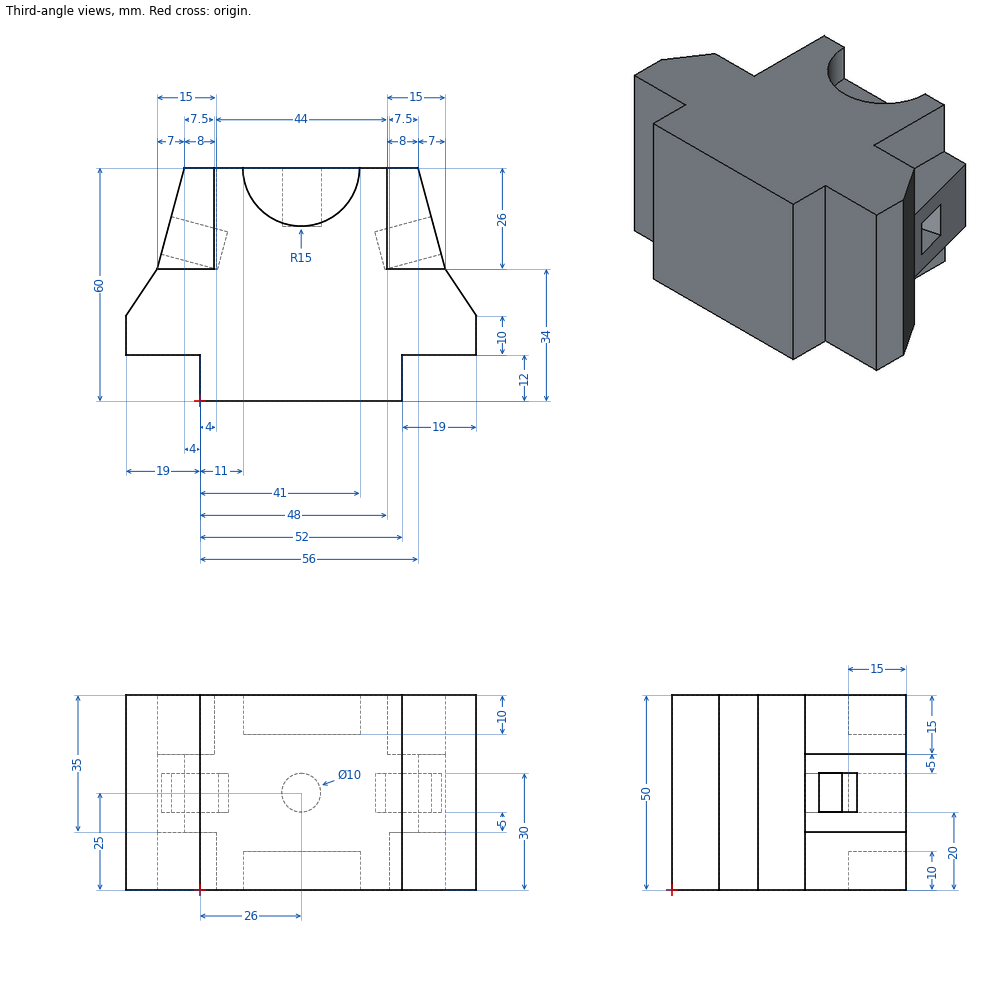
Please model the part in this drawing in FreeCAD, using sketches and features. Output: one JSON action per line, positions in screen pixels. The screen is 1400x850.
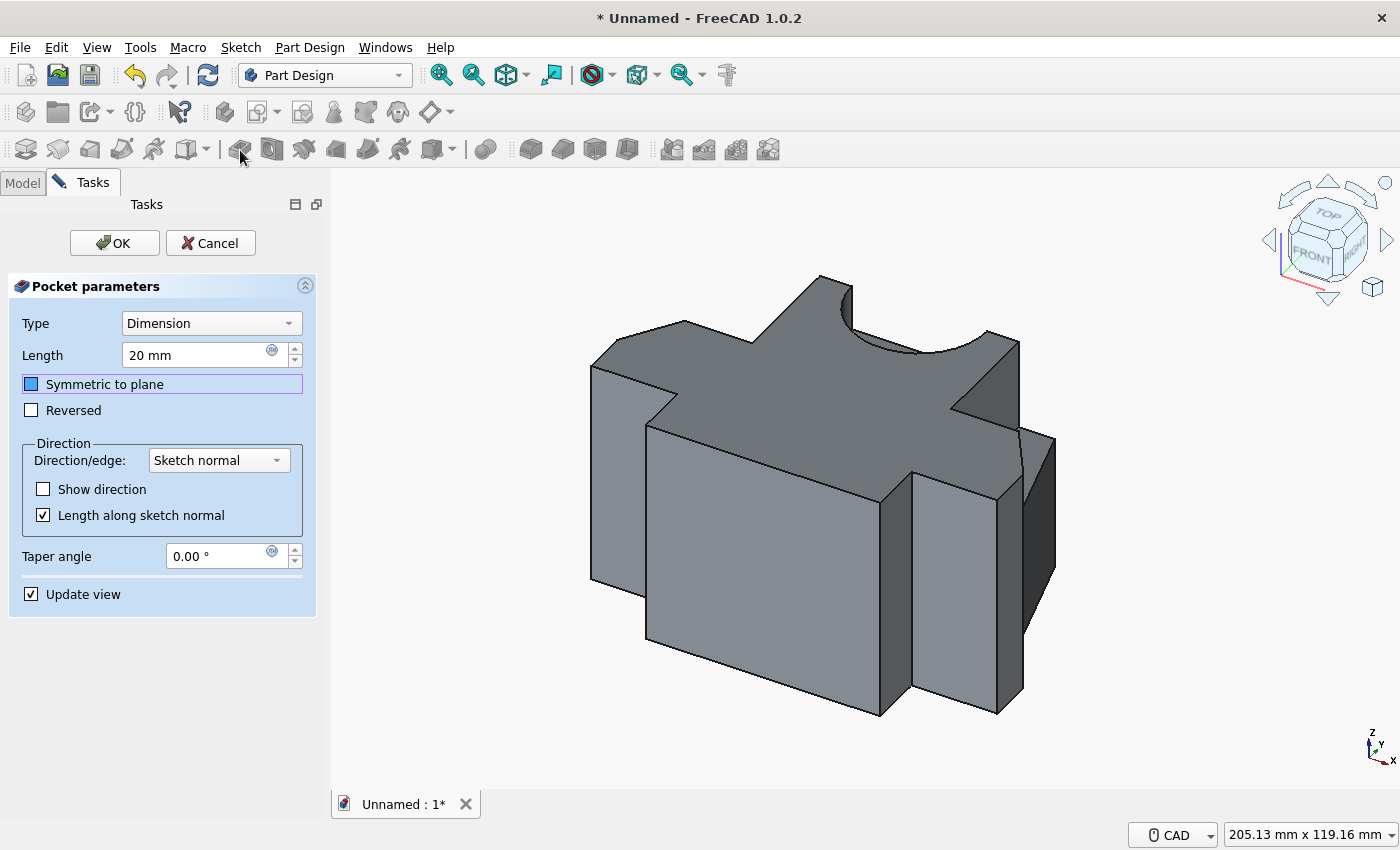
{"action": "left_click", "coordinate": [30, 410]}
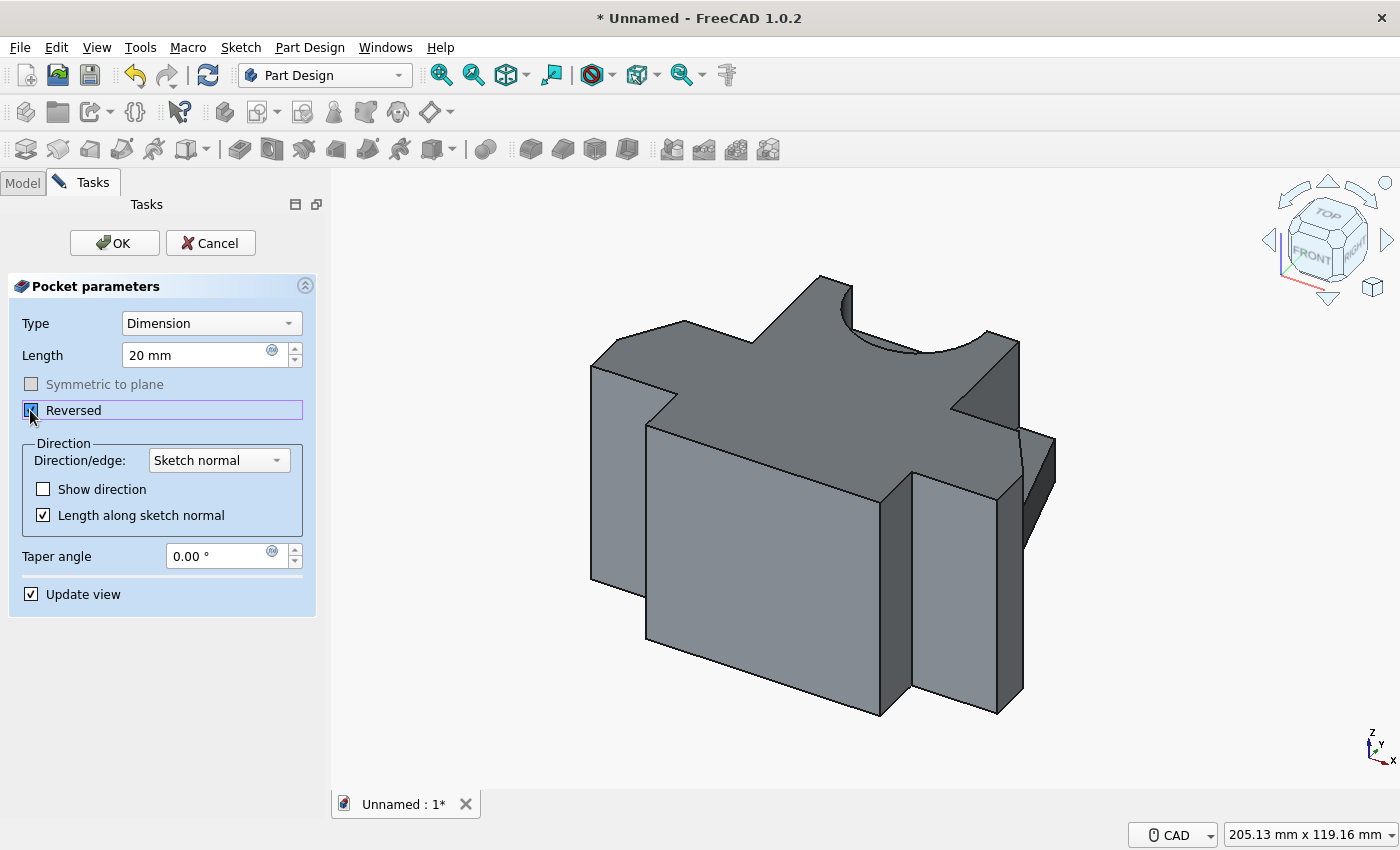
{"action": "left_click", "coordinate": [115, 243]}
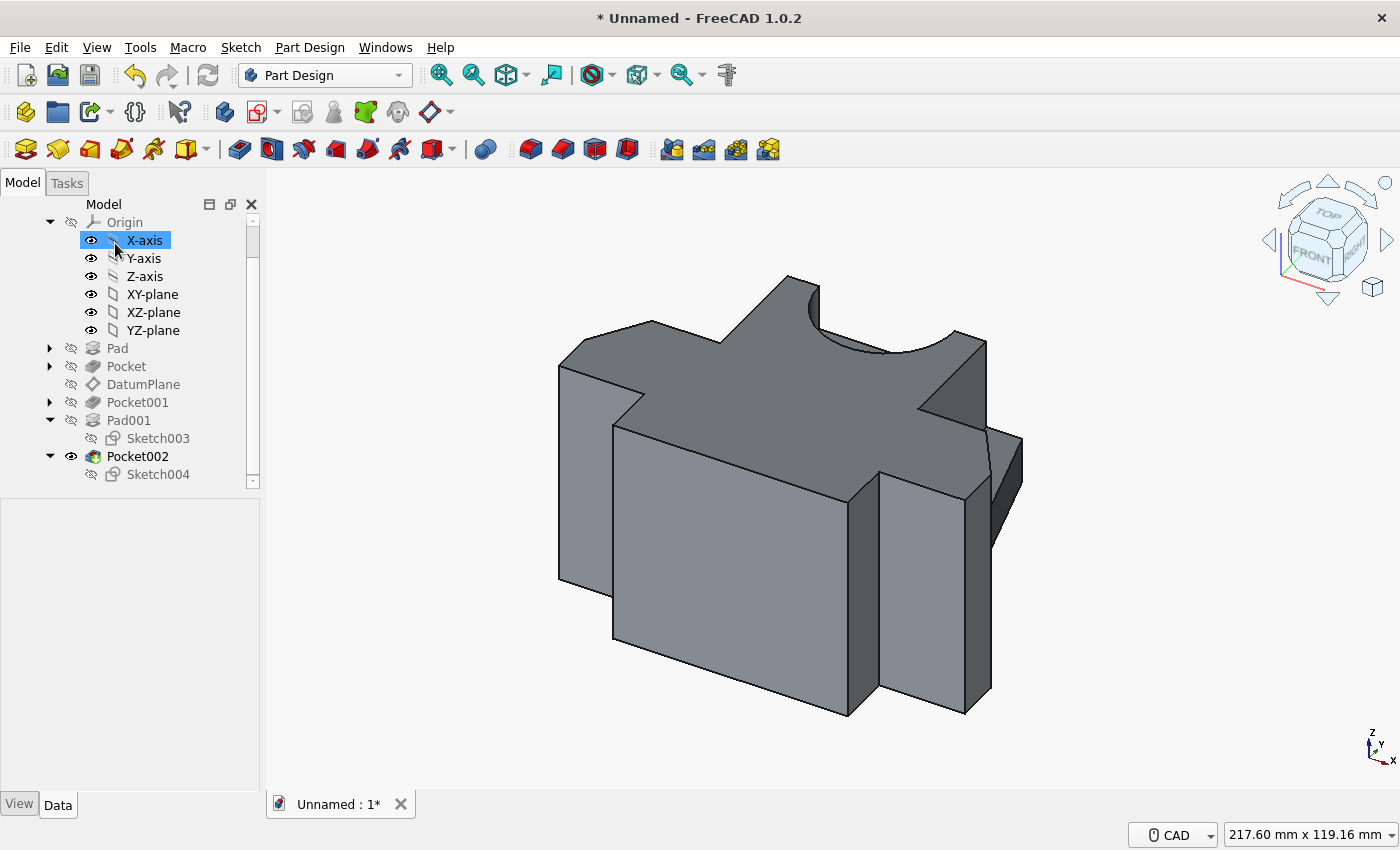
{"action": "key", "text": "5"}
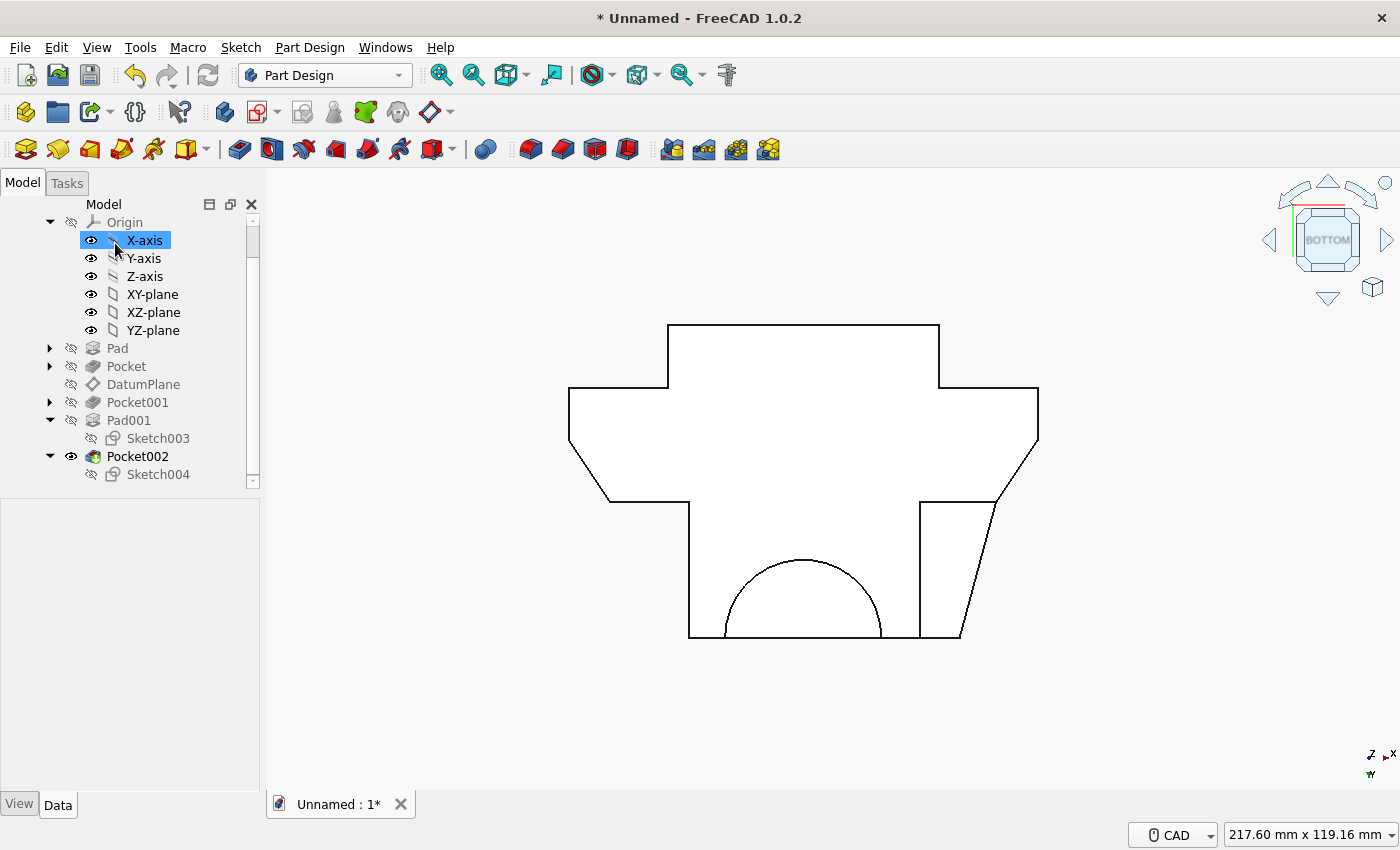
{"action": "left_click", "coordinate": [958, 530]}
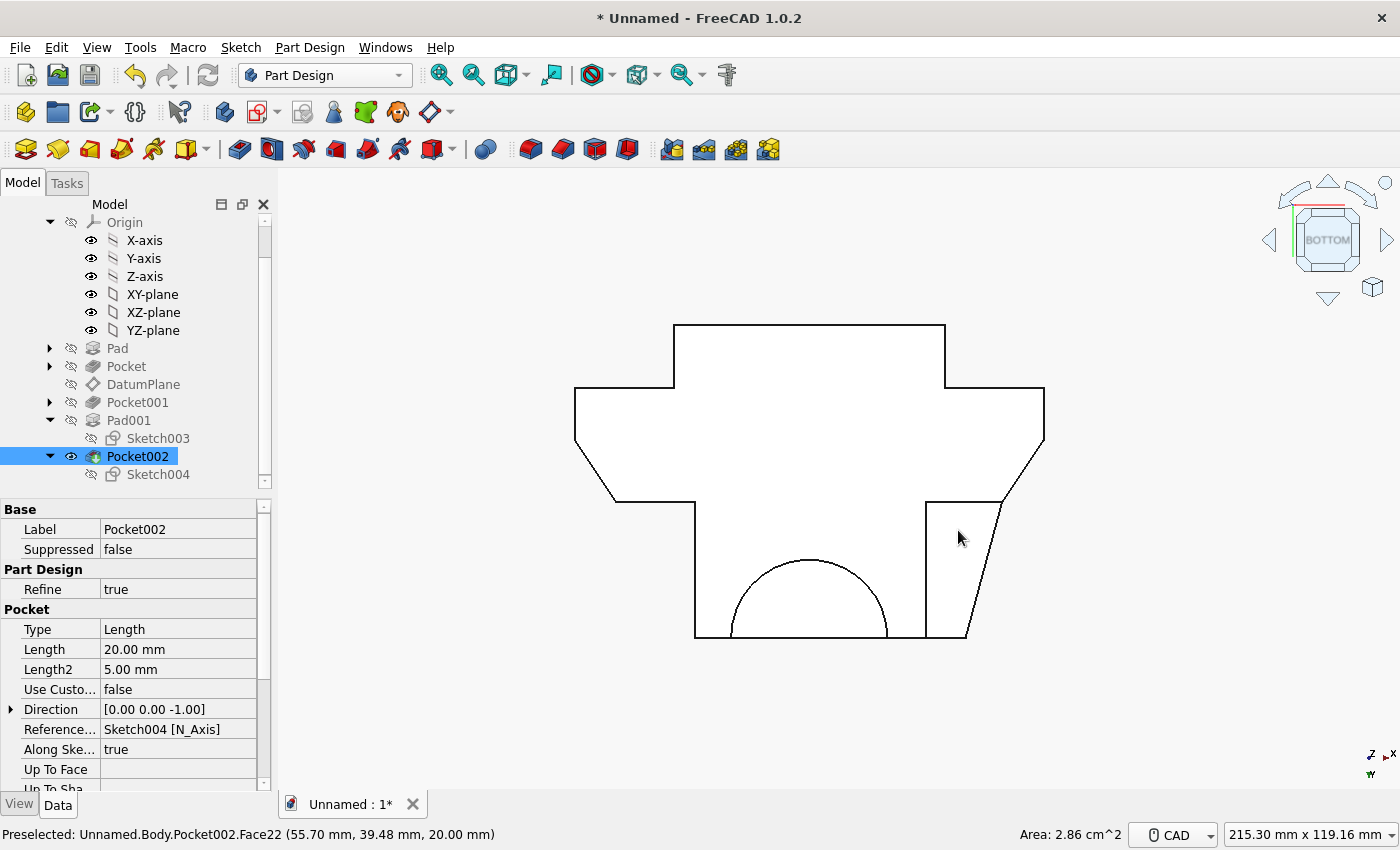
{"action": "left_click", "coordinate": [258, 112]}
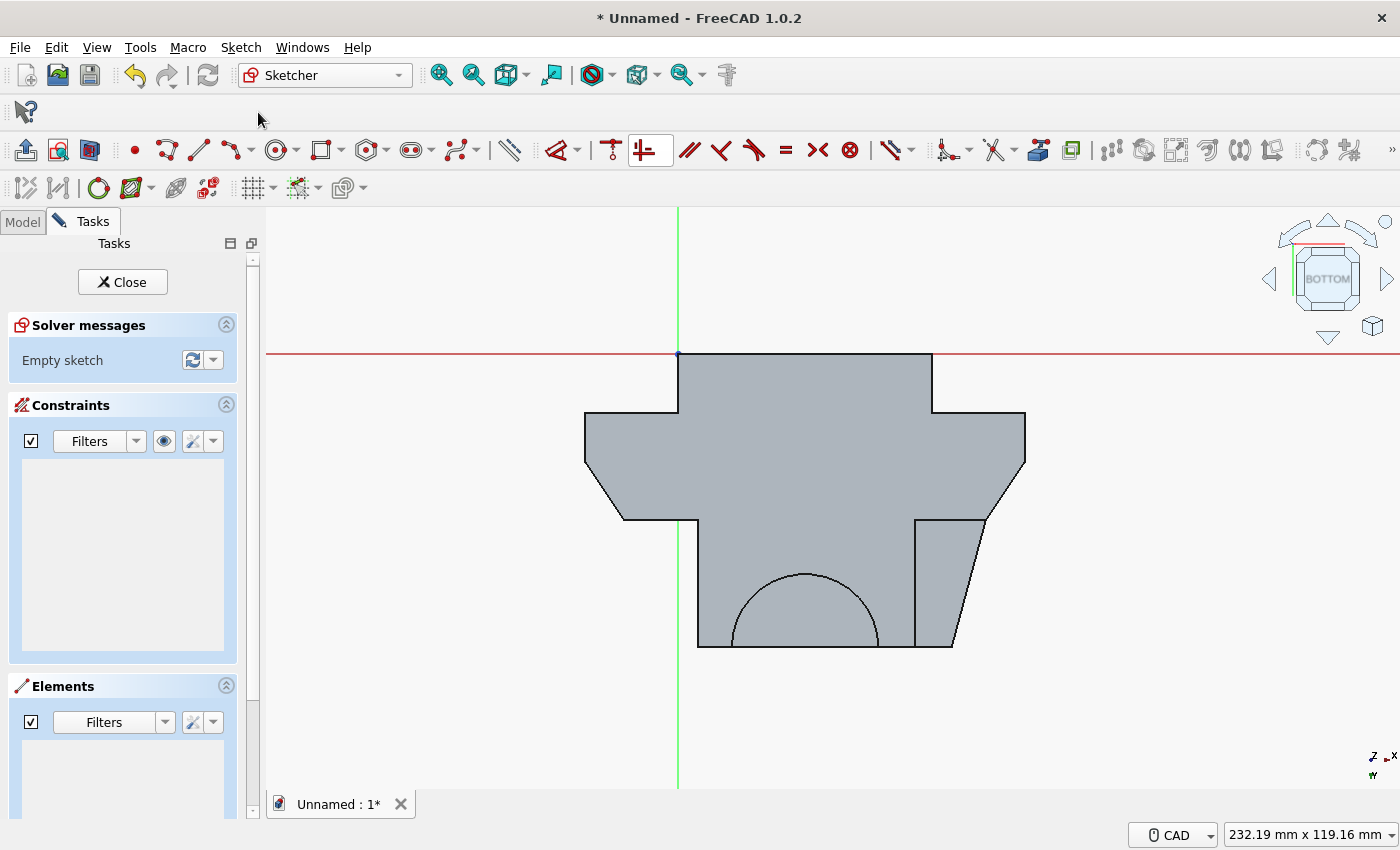
{"action": "left_click", "coordinate": [90, 150]}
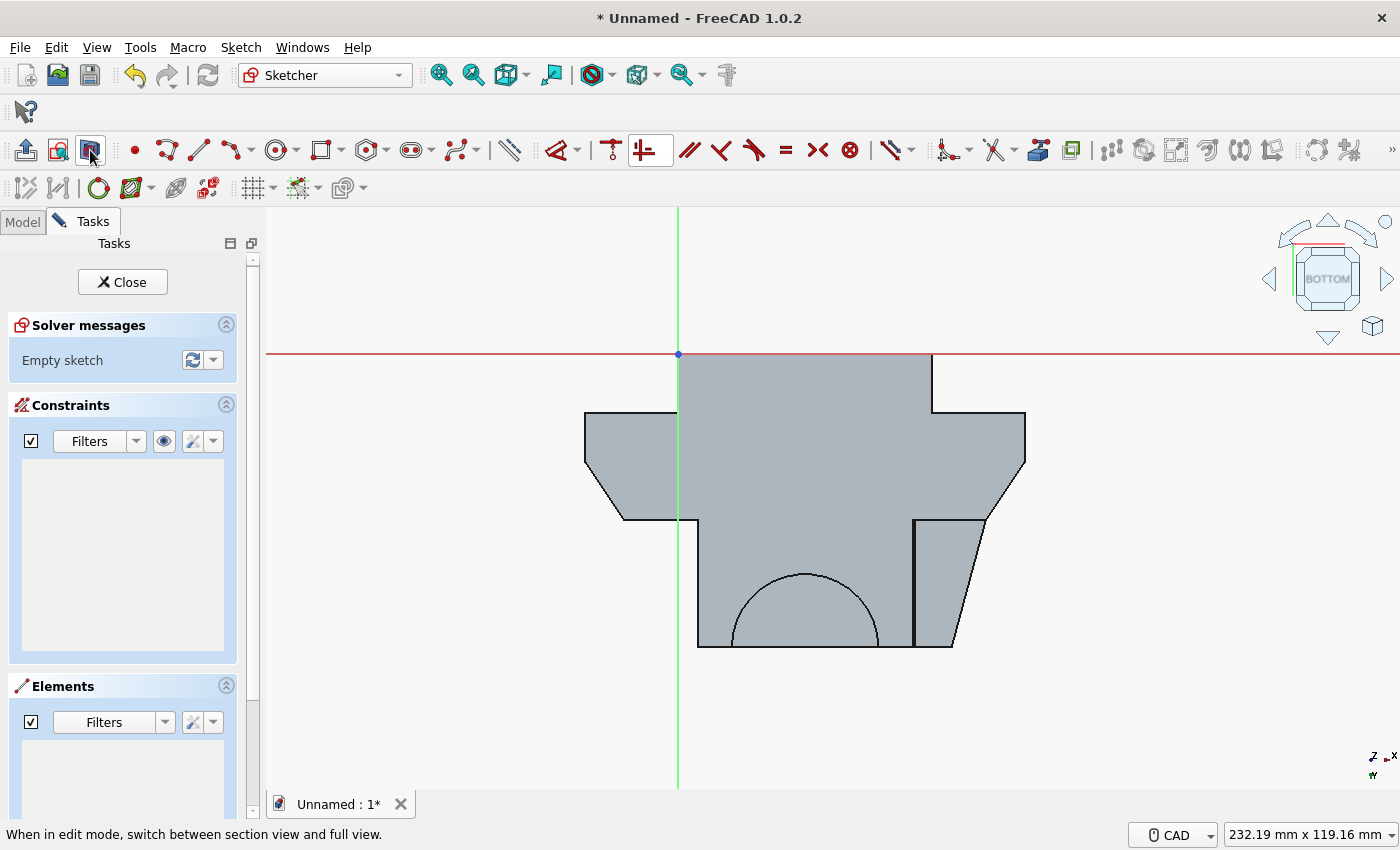
{"action": "left_click", "coordinate": [168, 150]}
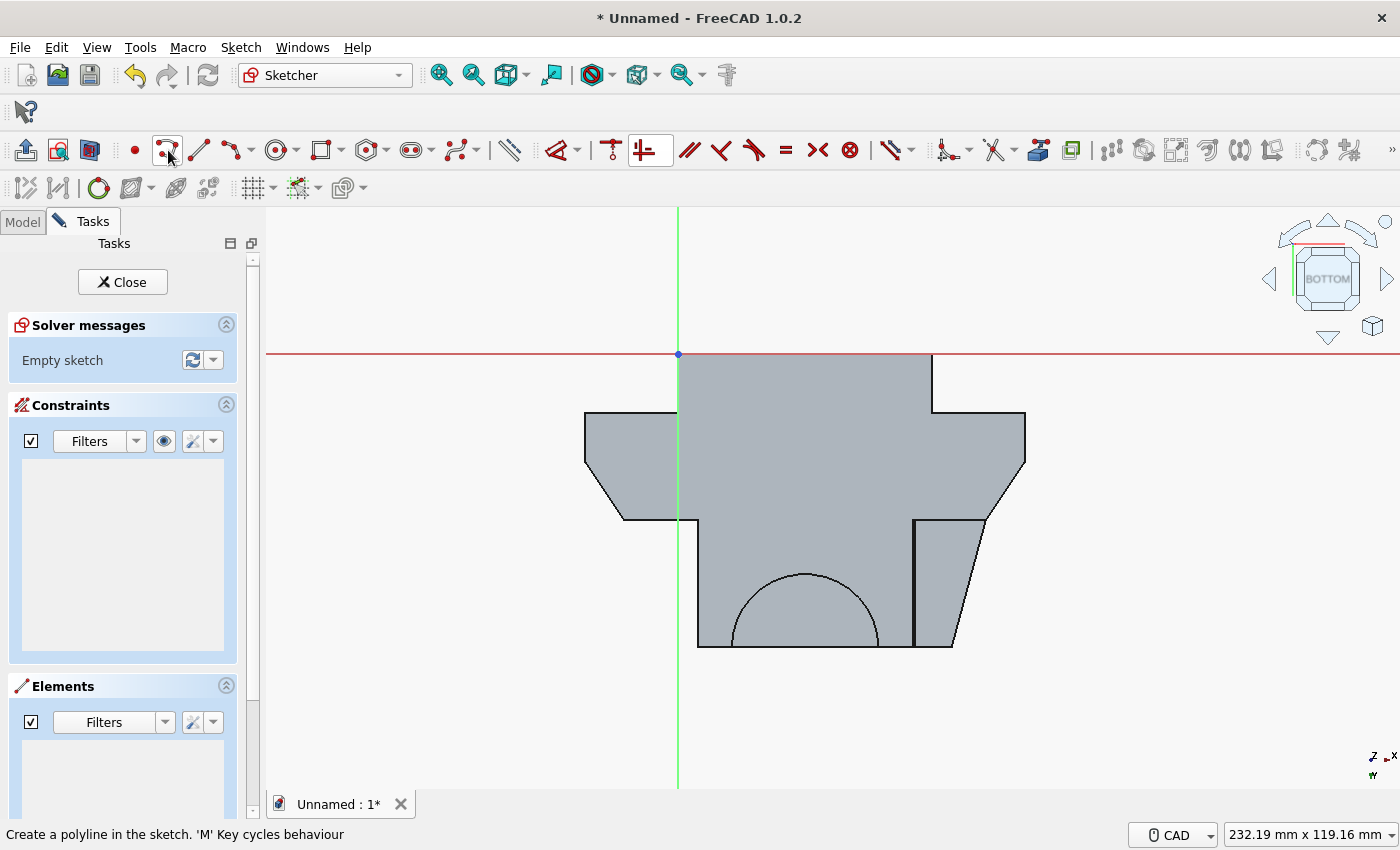
{"action": "left_click", "coordinate": [915, 520]}
{"action": "left_click", "coordinate": [915, 647]}
{"action": "left_click", "coordinate": [952, 647]}
{"action": "left_click", "coordinate": [986, 520]}
{"action": "left_click", "coordinate": [915, 521]}
{"action": "key", "text": "Escape"}
{"action": "key", "text": "Escape"}